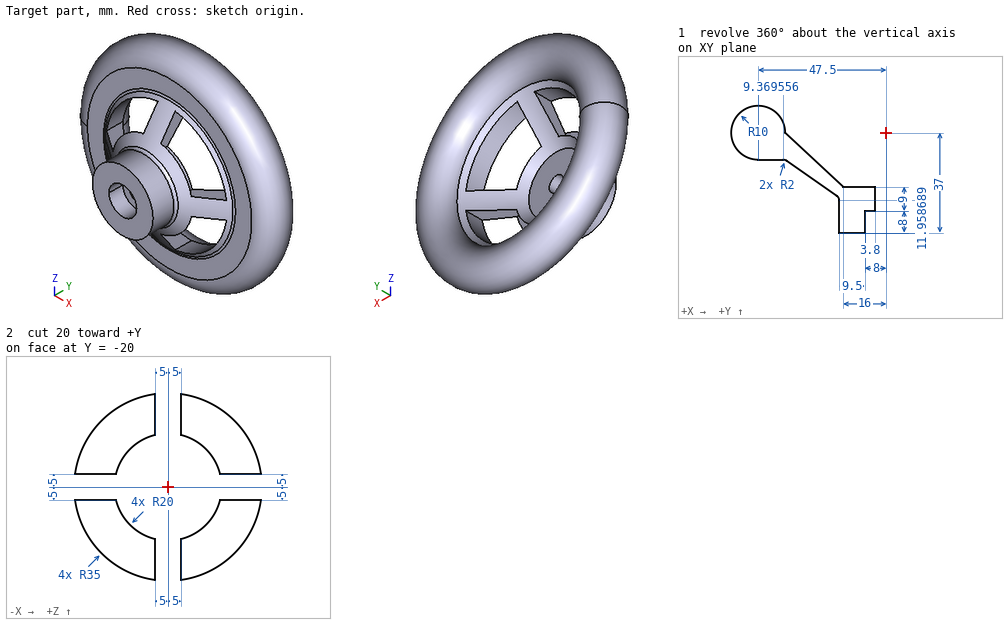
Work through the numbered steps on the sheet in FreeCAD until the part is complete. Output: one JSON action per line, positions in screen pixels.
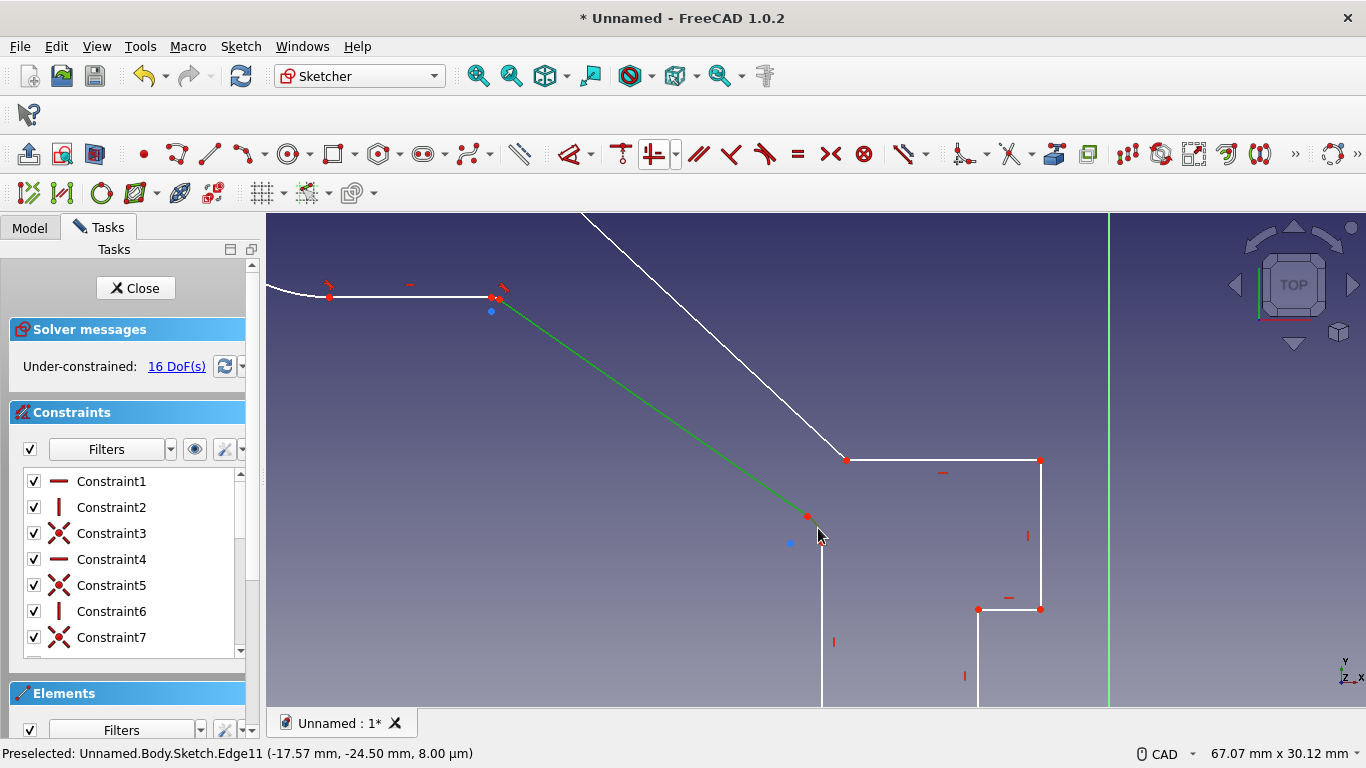
{"action": "key", "text": "t"}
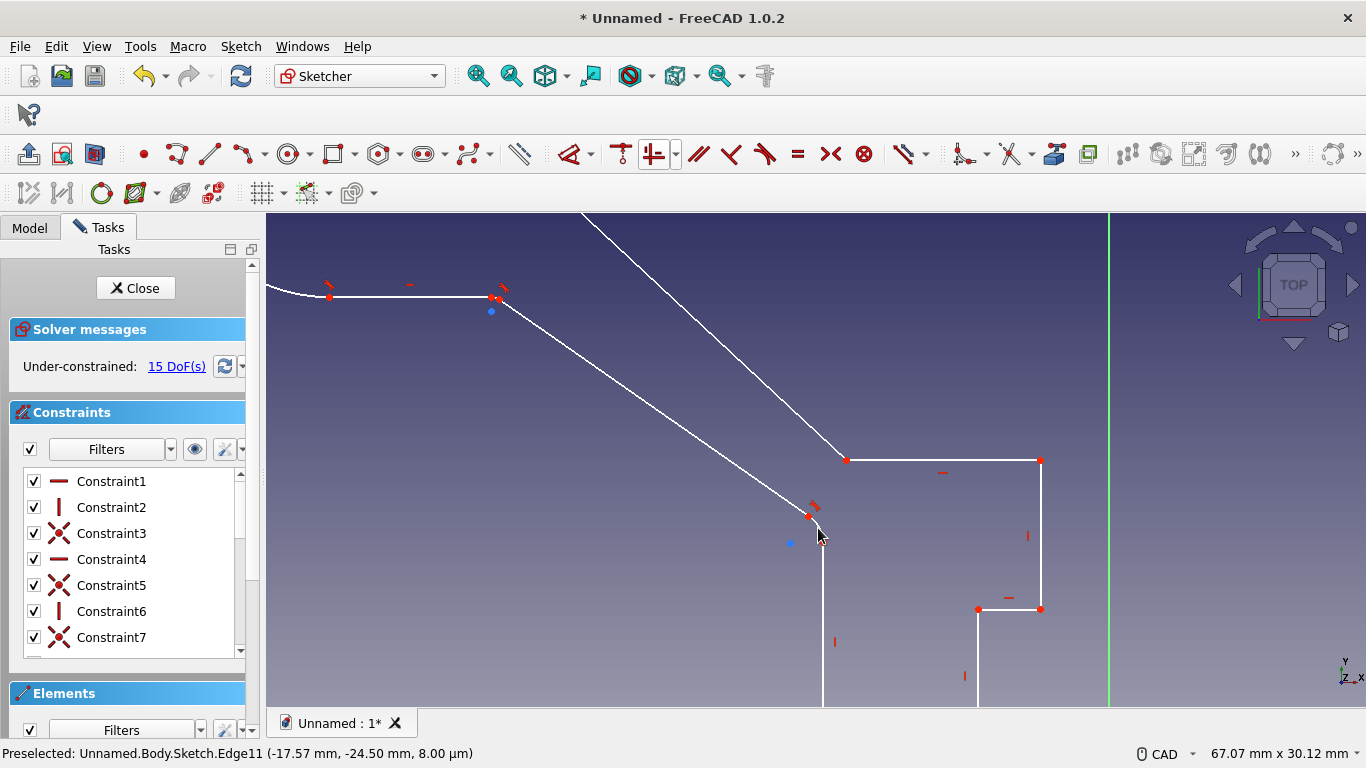
{"action": "left_click", "coordinate": [823, 602]}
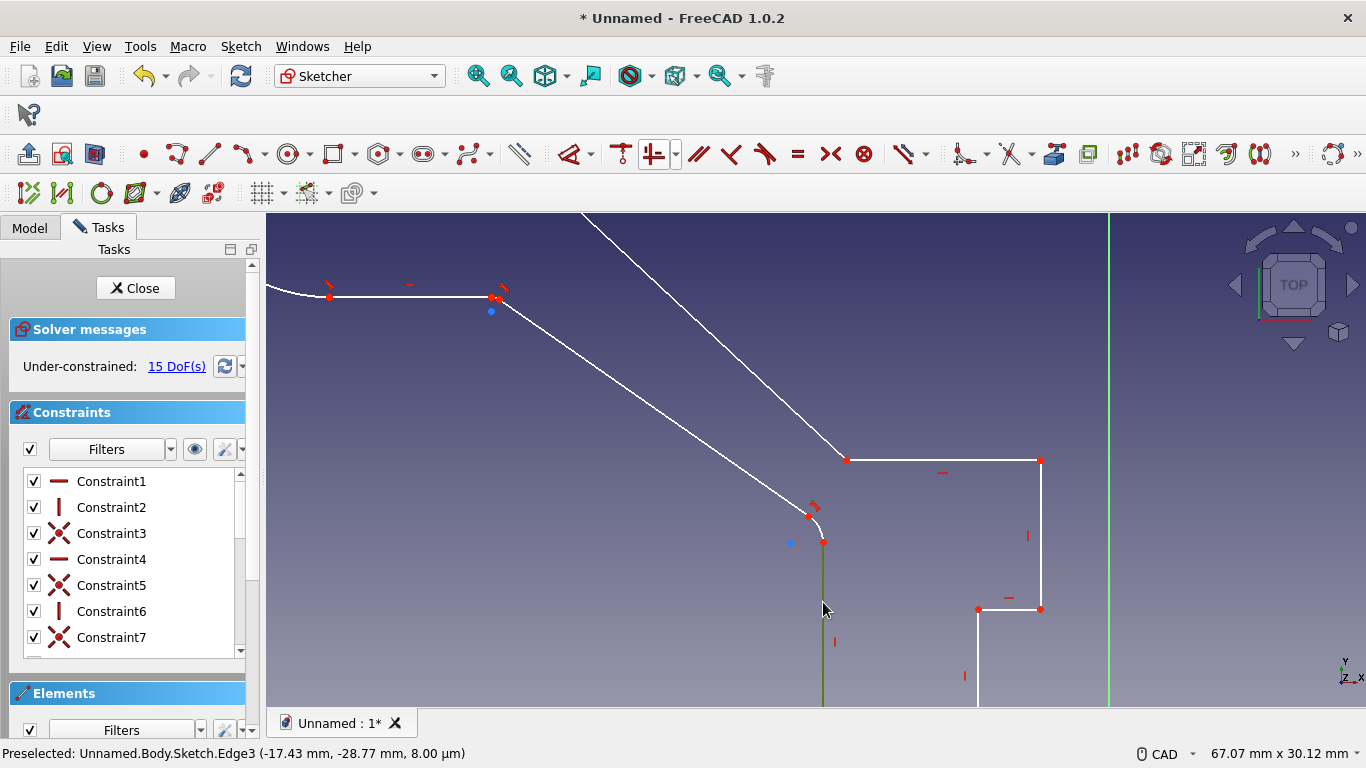
{"action": "scroll", "coordinate": [822, 534], "scroll_direction": "up", "scroll_amount": 2}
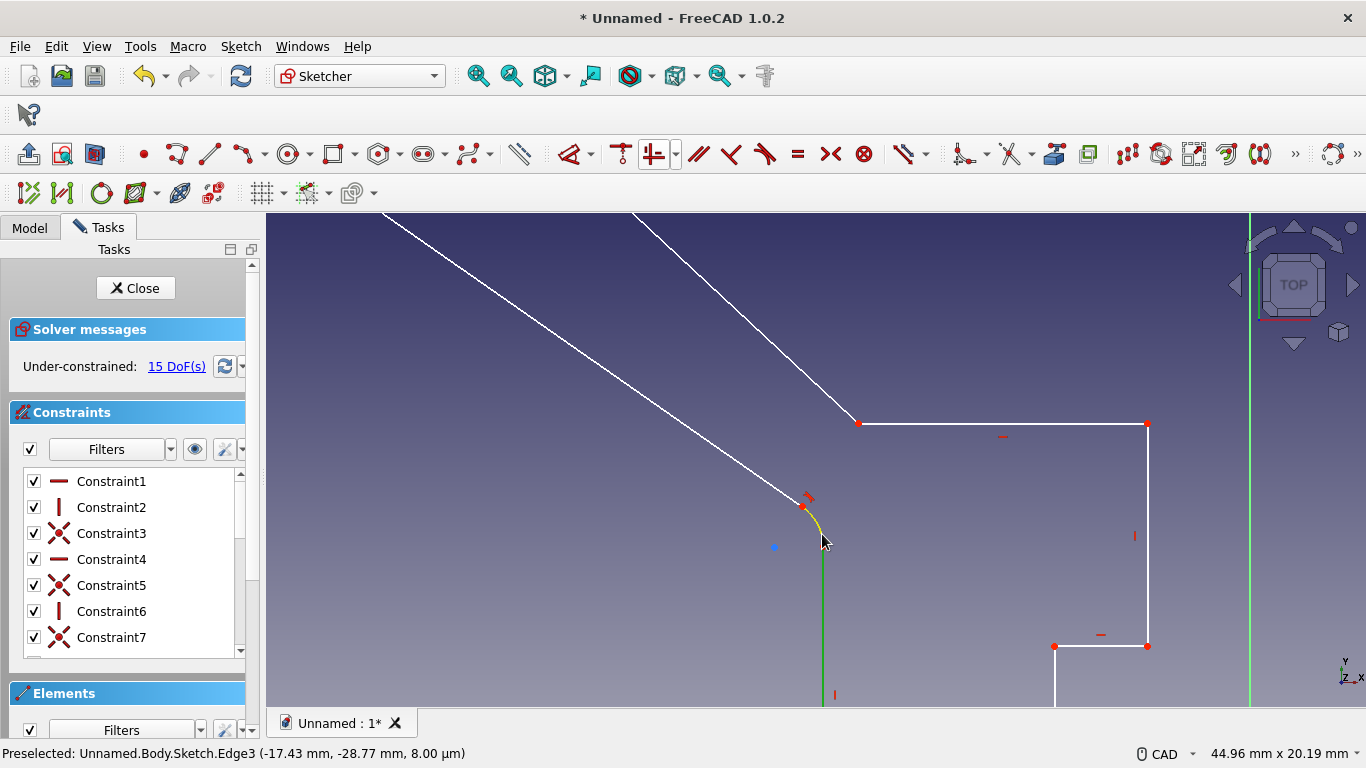
{"action": "left_click", "coordinate": [821, 533]}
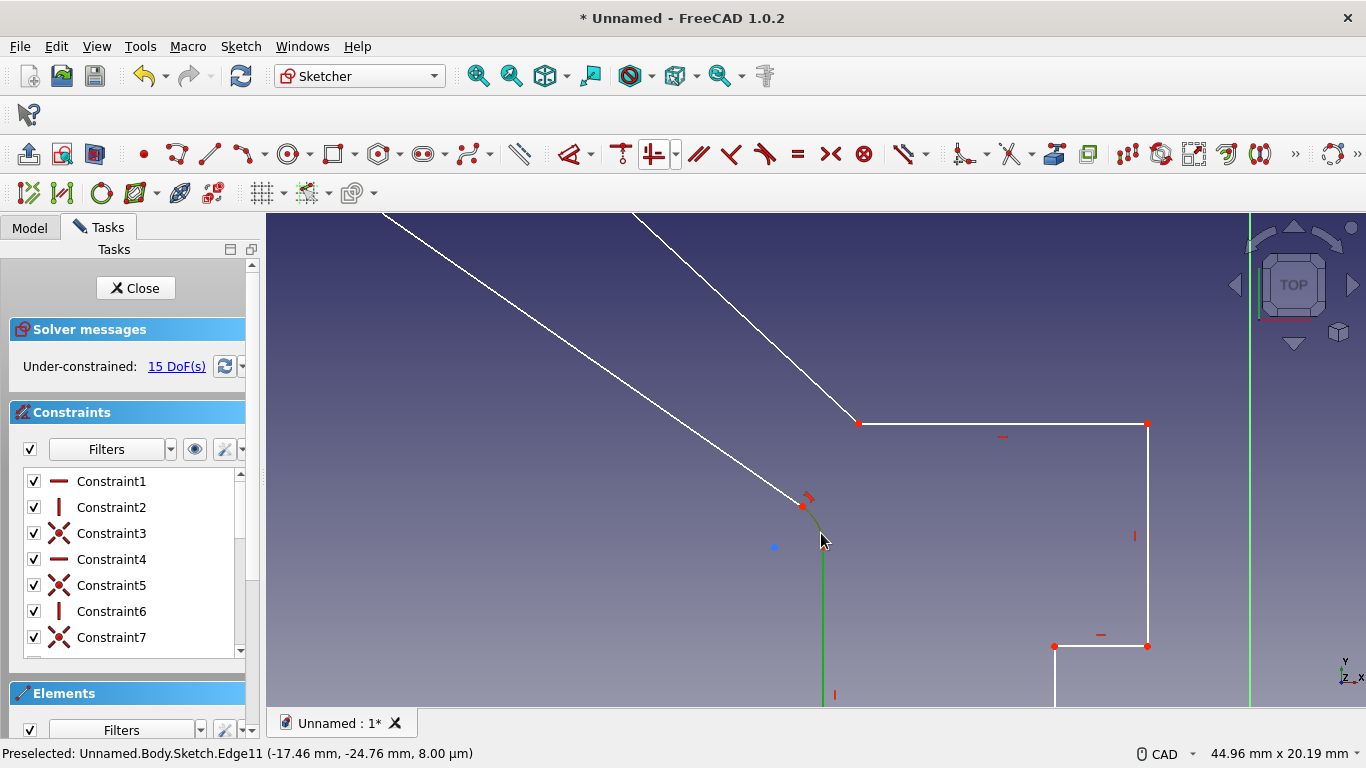
{"action": "key", "text": "t"}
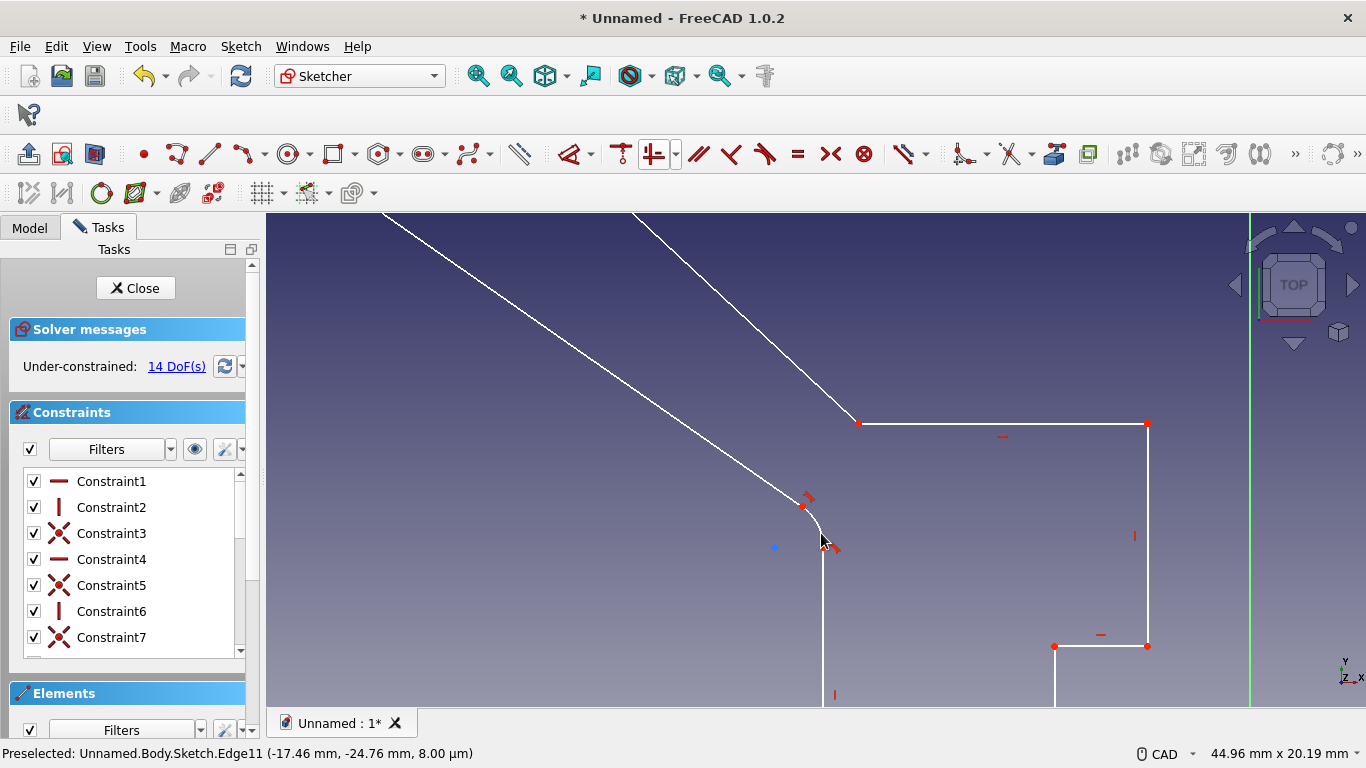
{"action": "scroll", "coordinate": [819, 529], "scroll_direction": "down", "scroll_amount": 6}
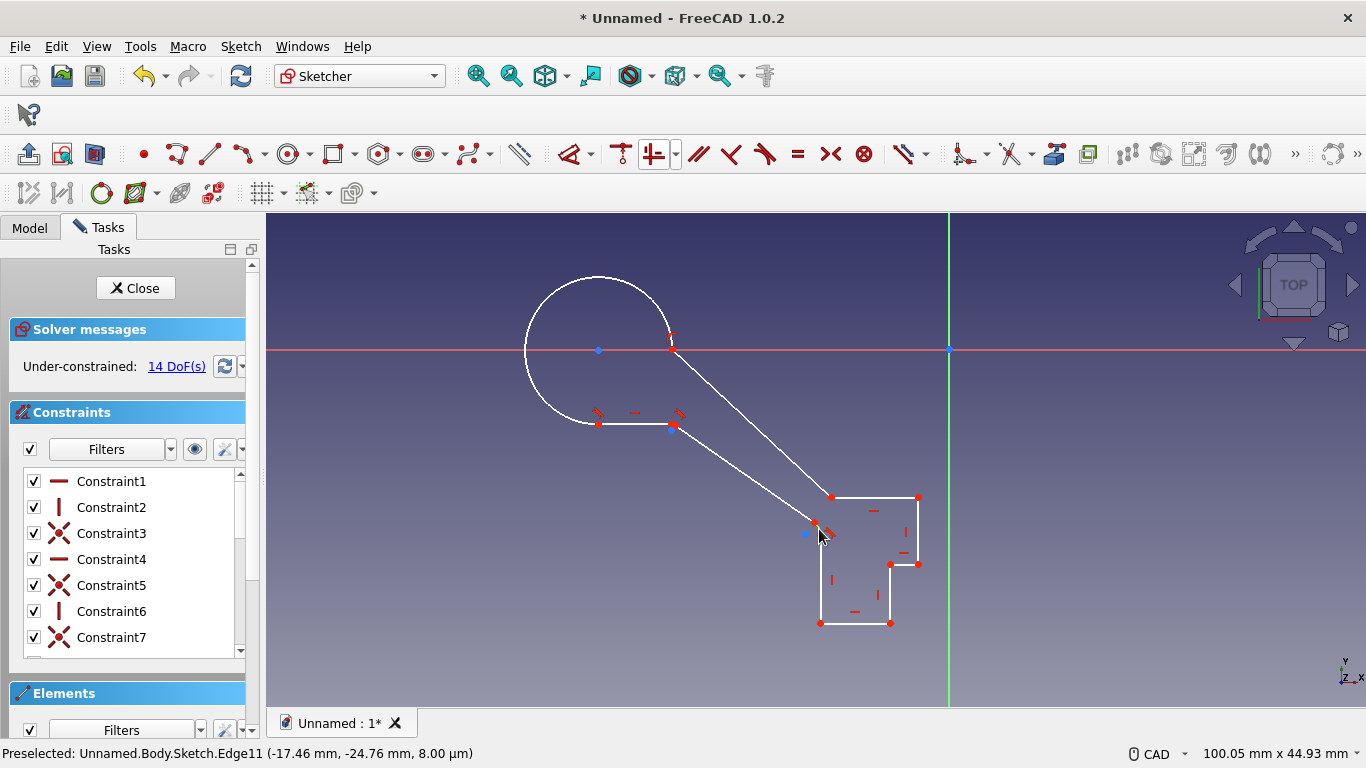
{"action": "scroll", "coordinate": [674, 425], "scroll_direction": "up", "scroll_amount": 10}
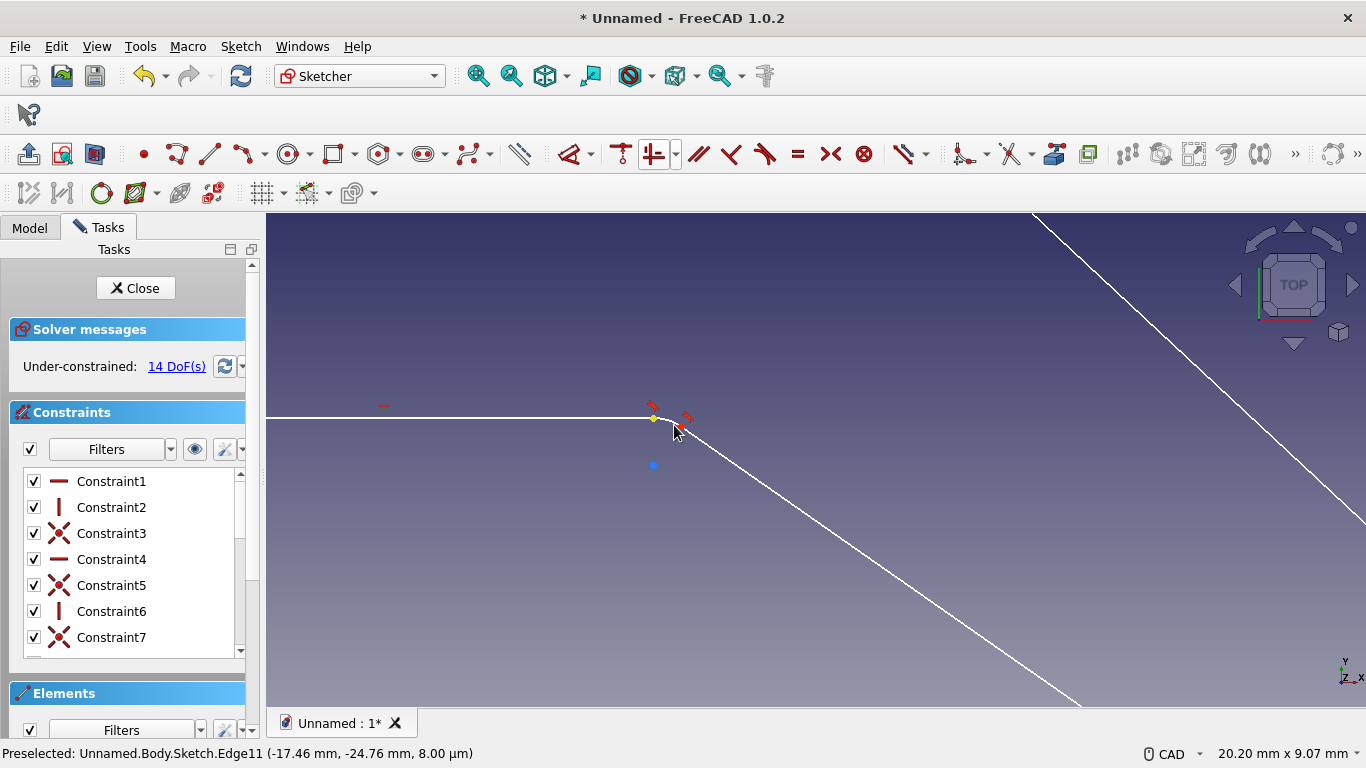
{"action": "left_click", "coordinate": [668, 420]}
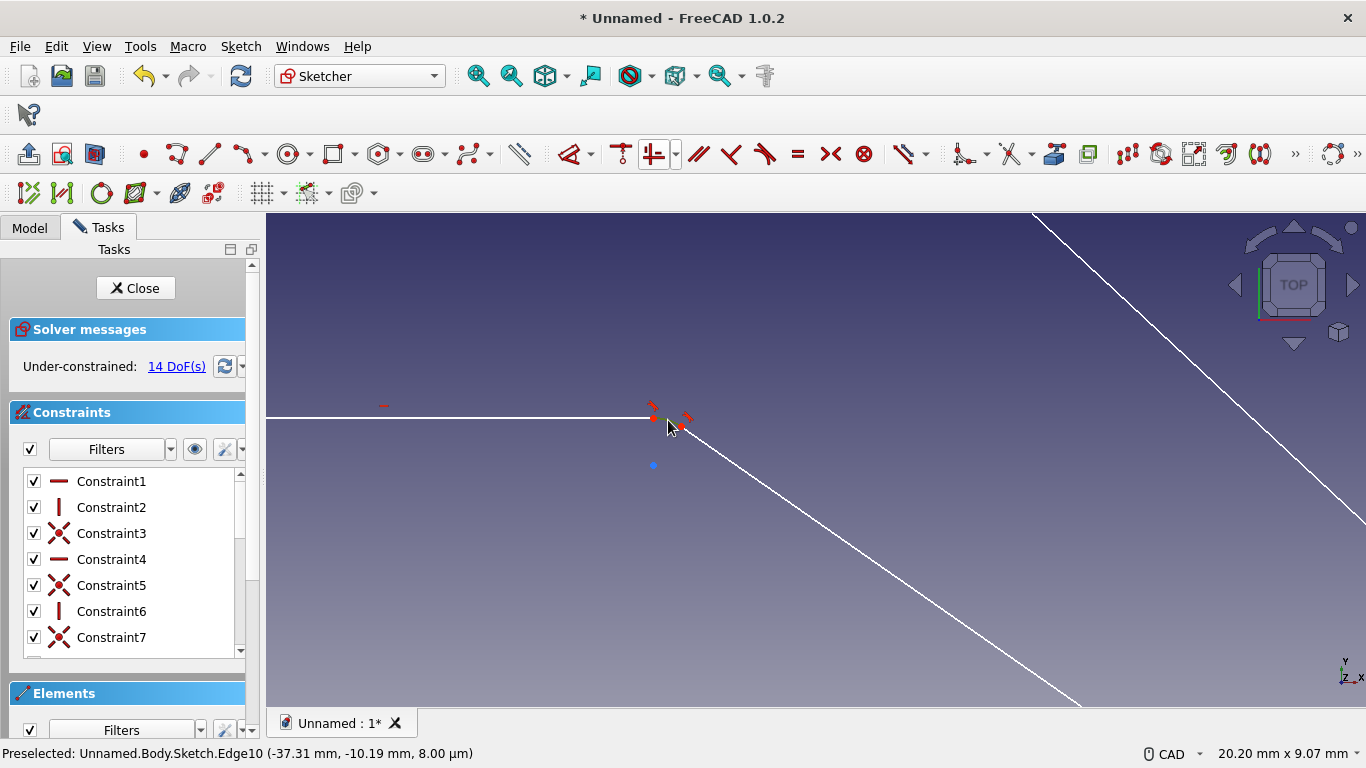
{"action": "scroll", "coordinate": [674, 425], "scroll_direction": "down", "scroll_amount": 10}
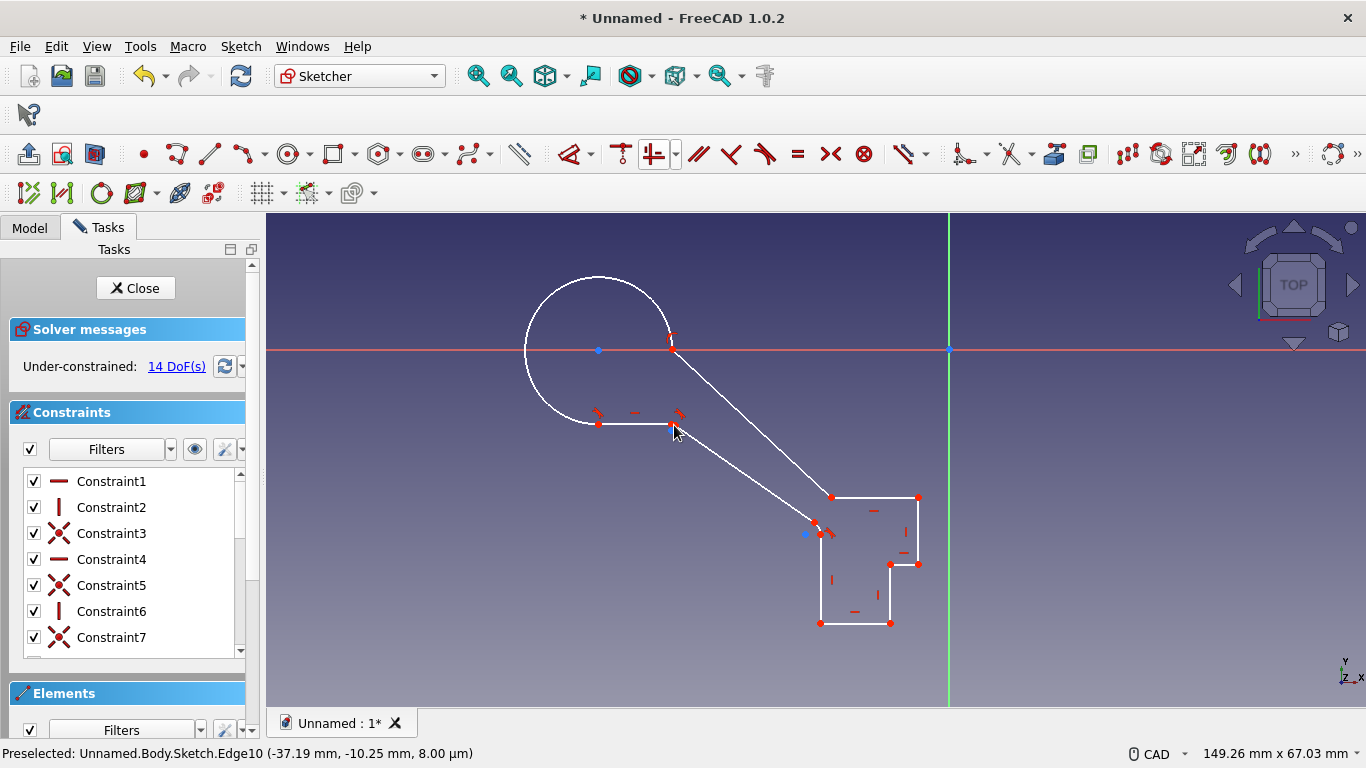
{"action": "scroll", "coordinate": [820, 531], "scroll_direction": "up", "scroll_amount": 6}